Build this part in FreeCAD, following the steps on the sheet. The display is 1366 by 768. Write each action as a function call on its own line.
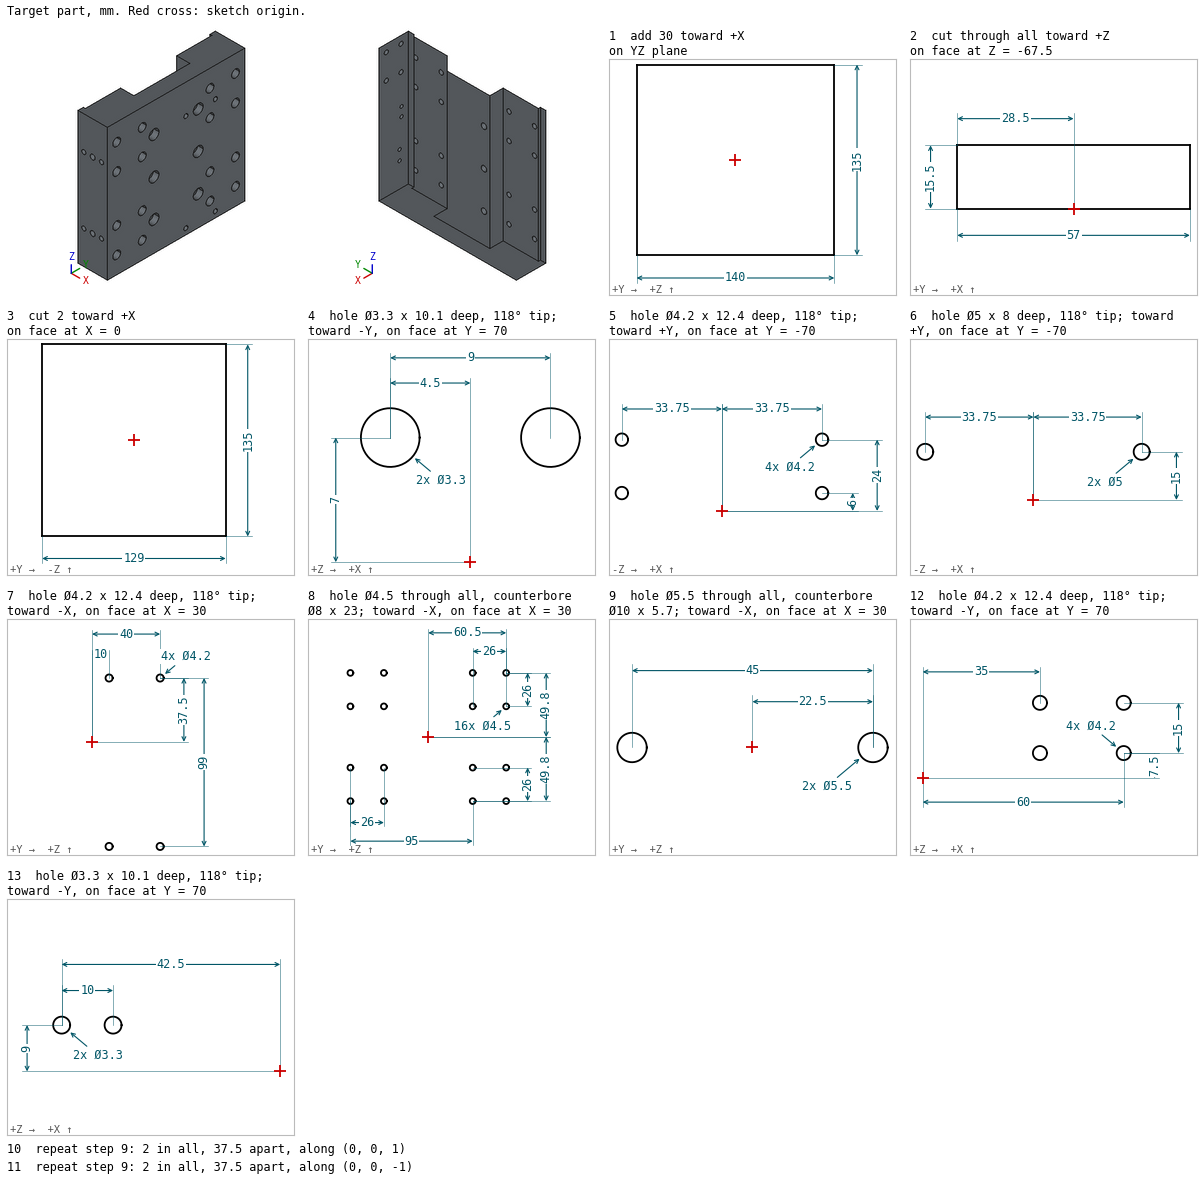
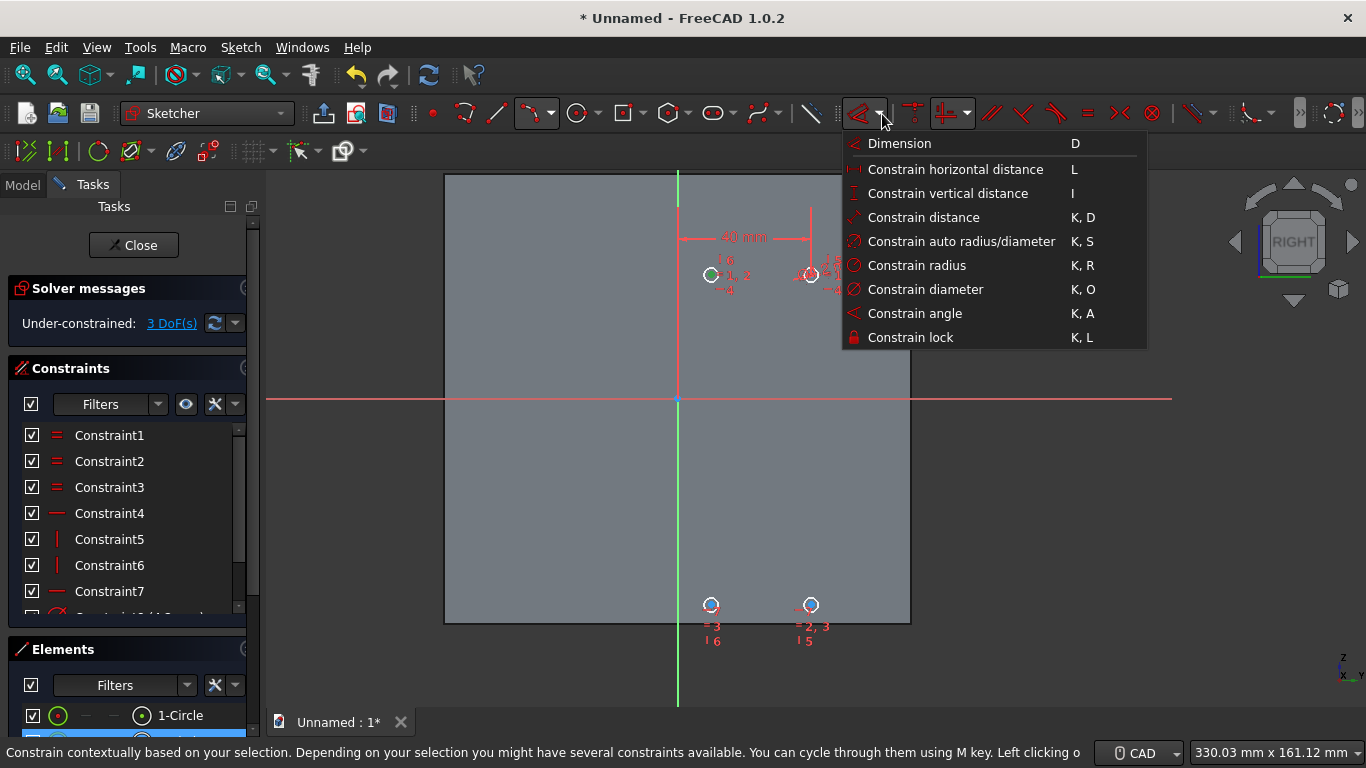
click(995, 169)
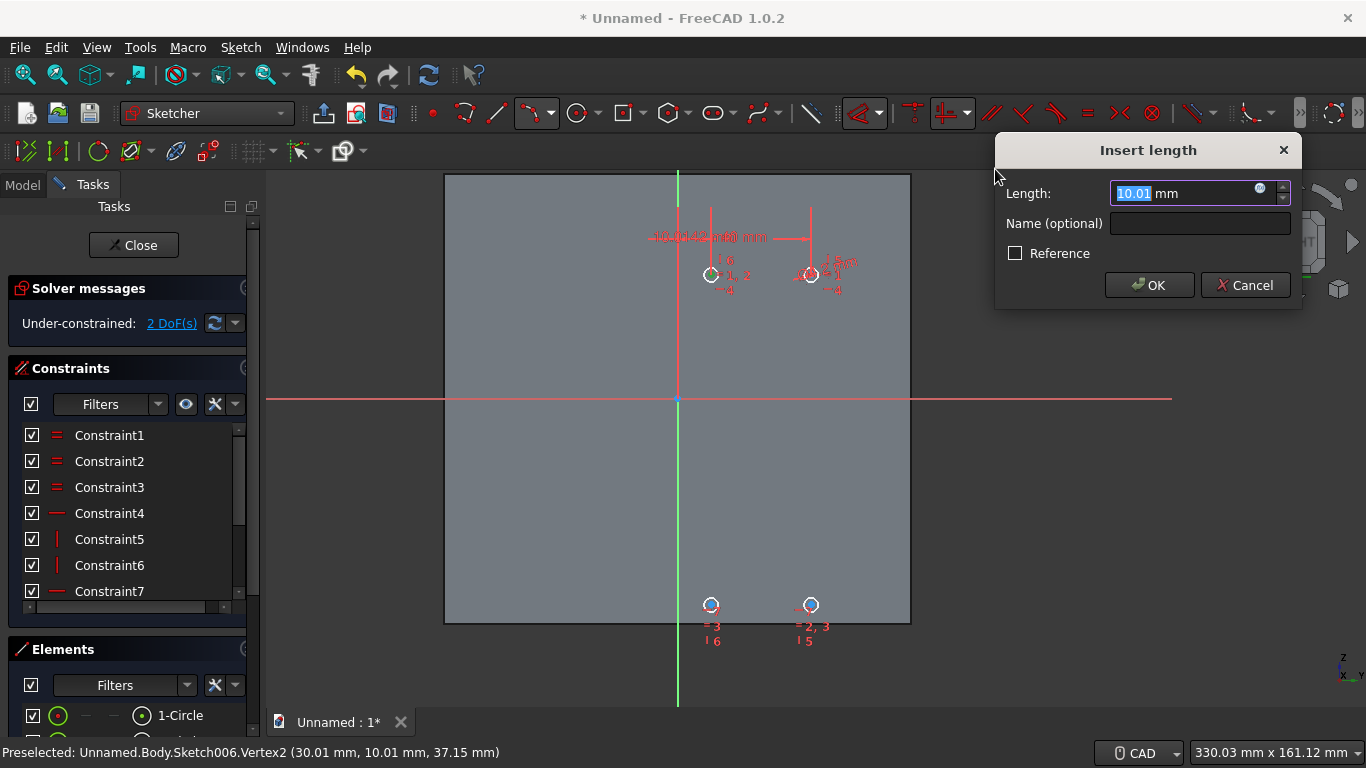
text(10)
key(Return)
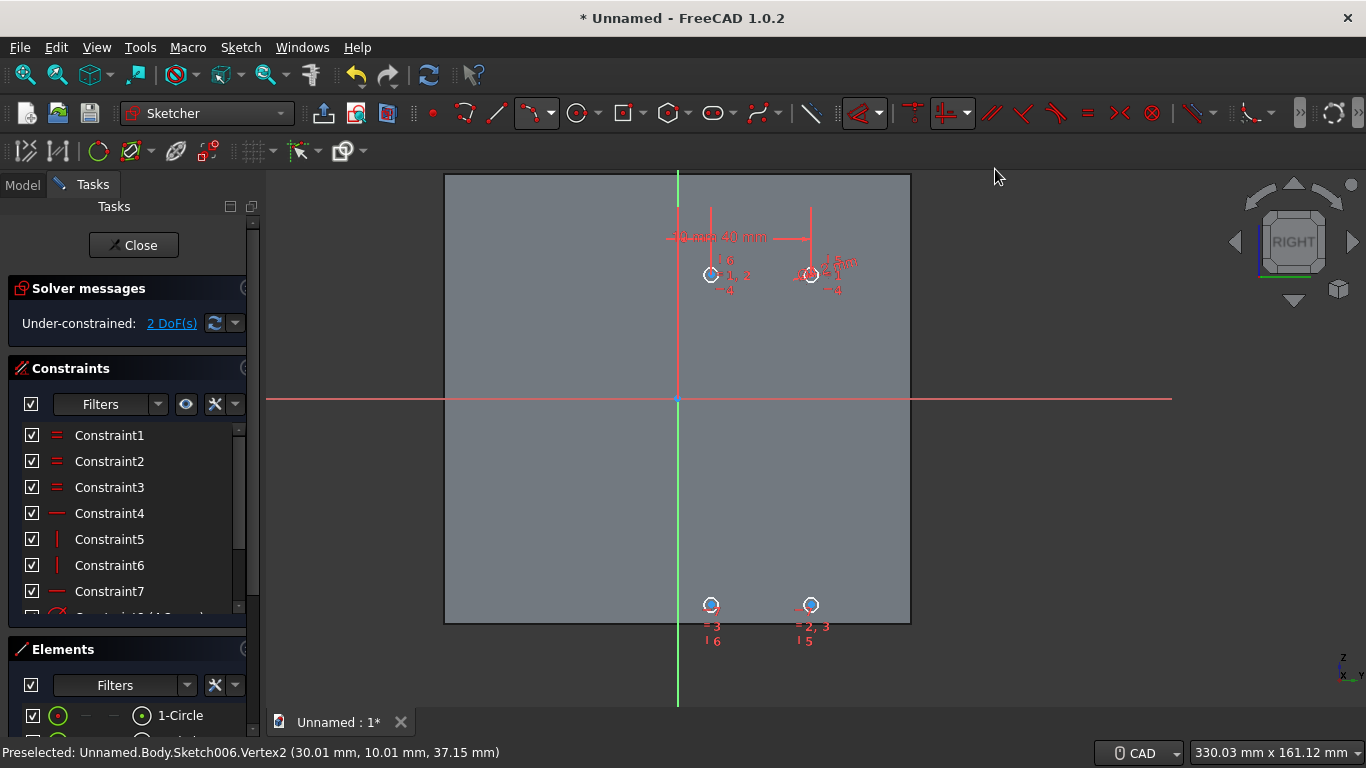
click(811, 275)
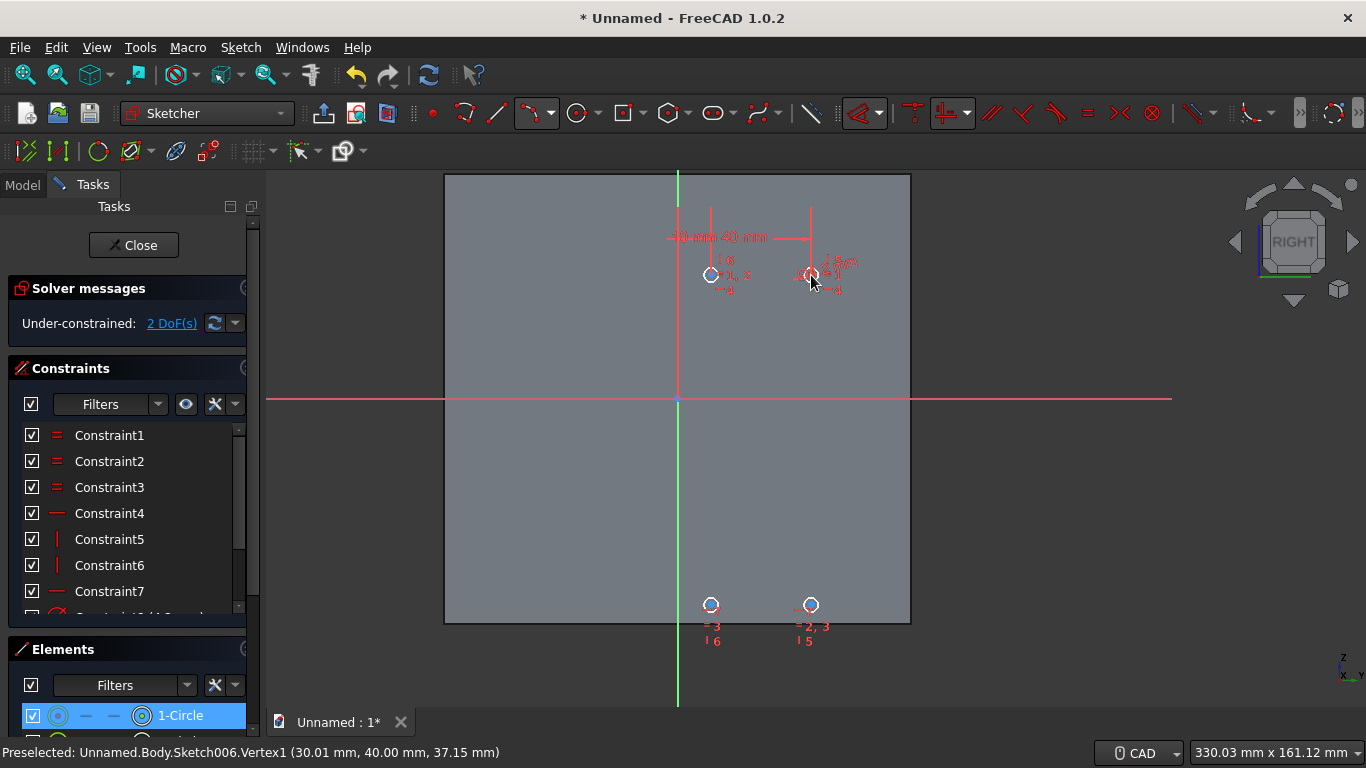
click(811, 605)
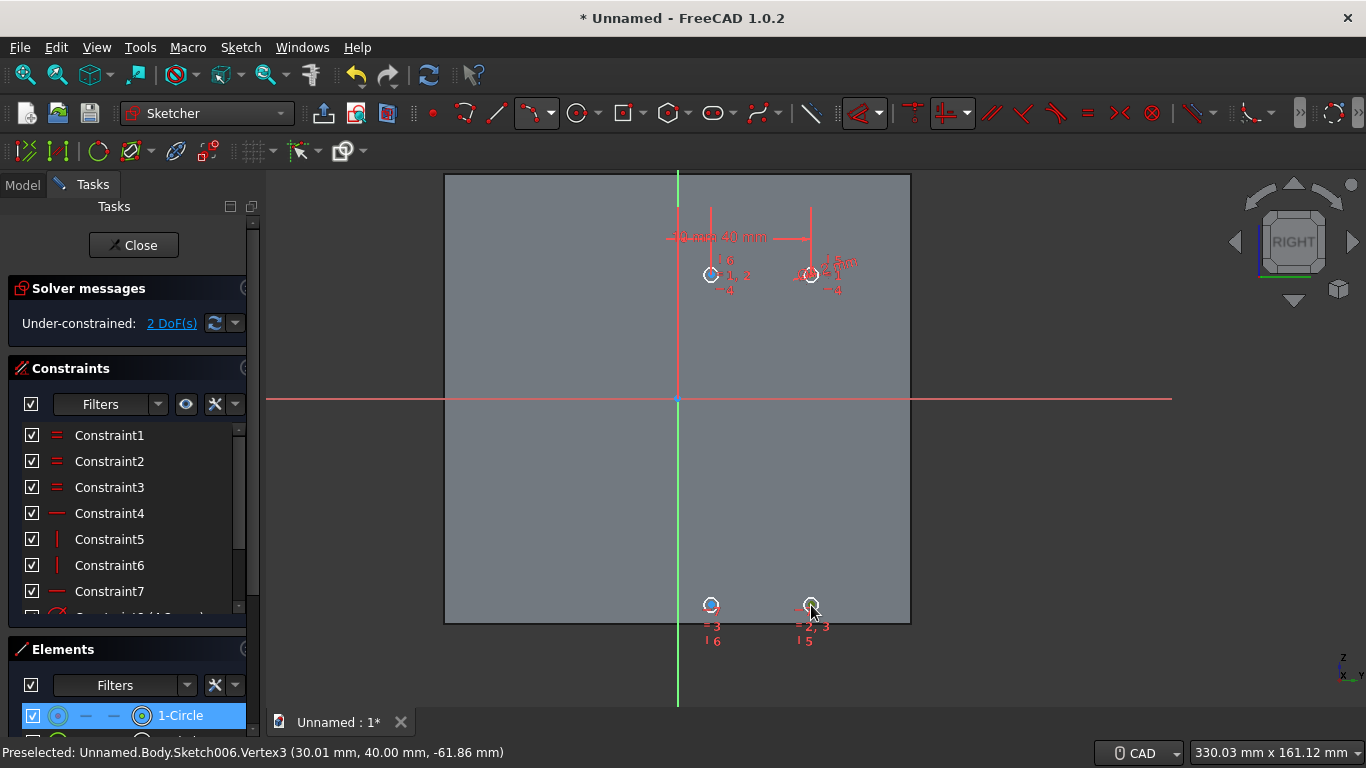
key(i)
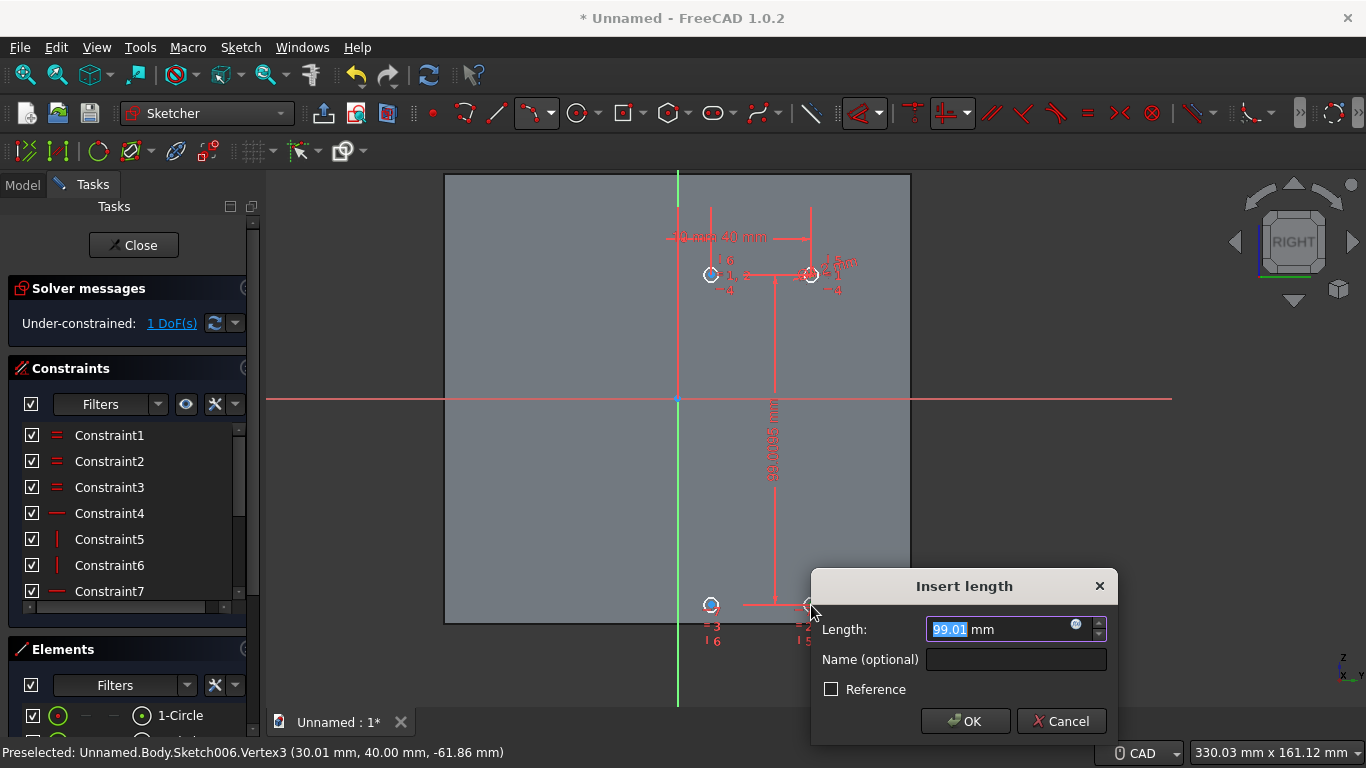
text(99)
key(Return)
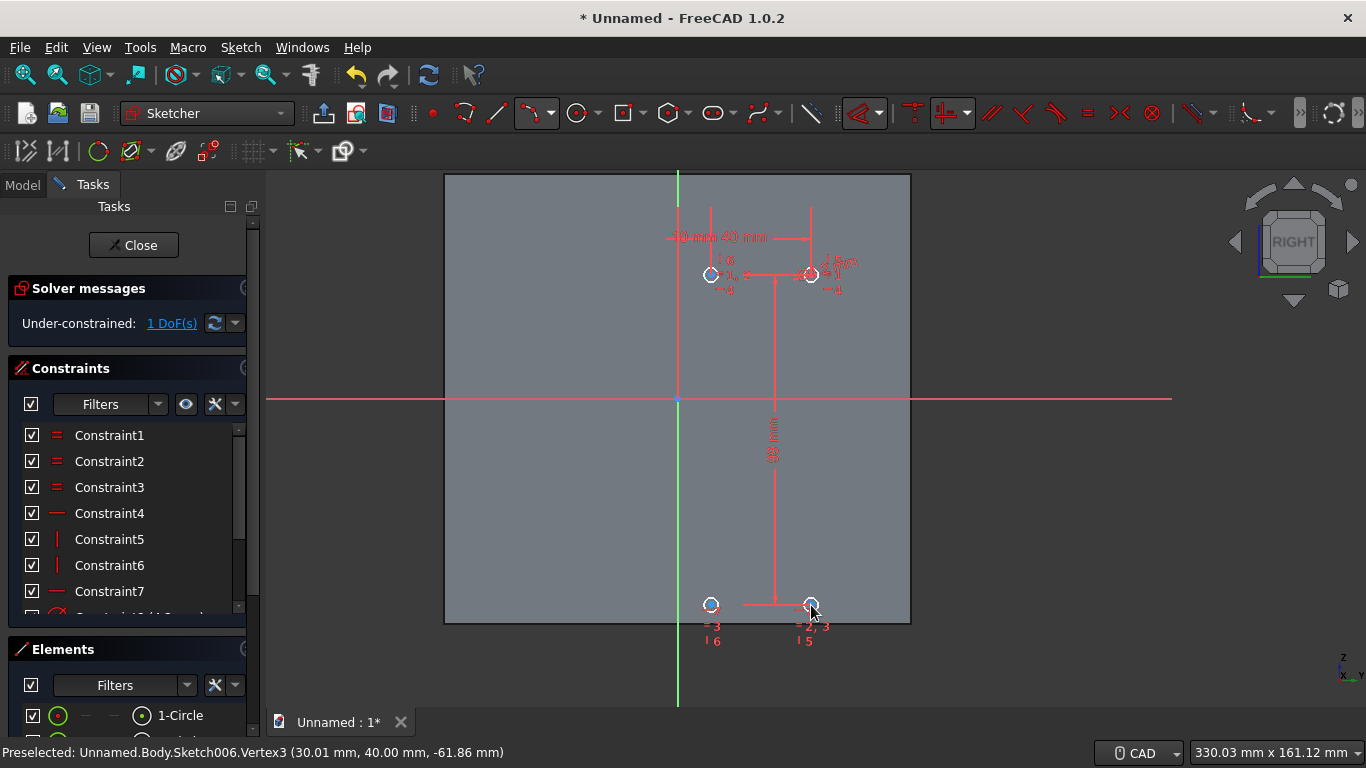
click(811, 275)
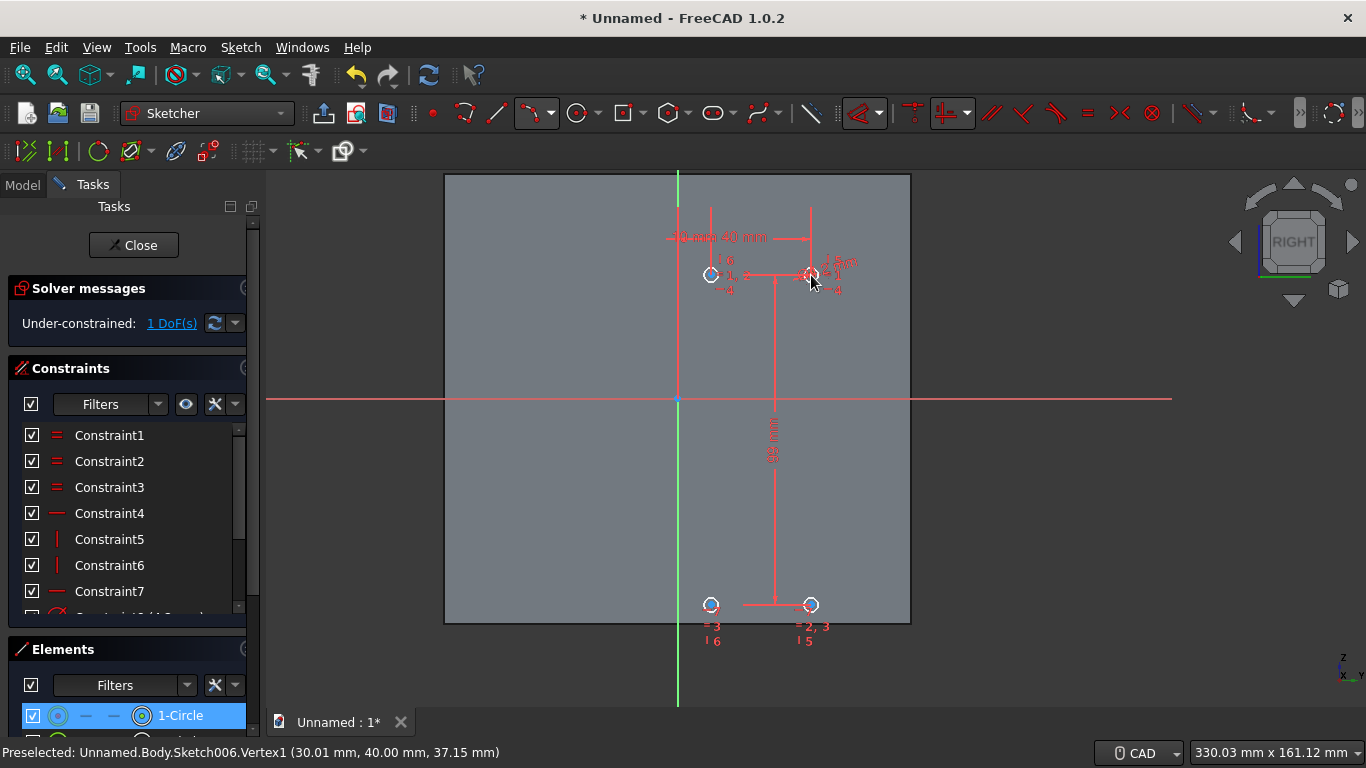
click(882, 114)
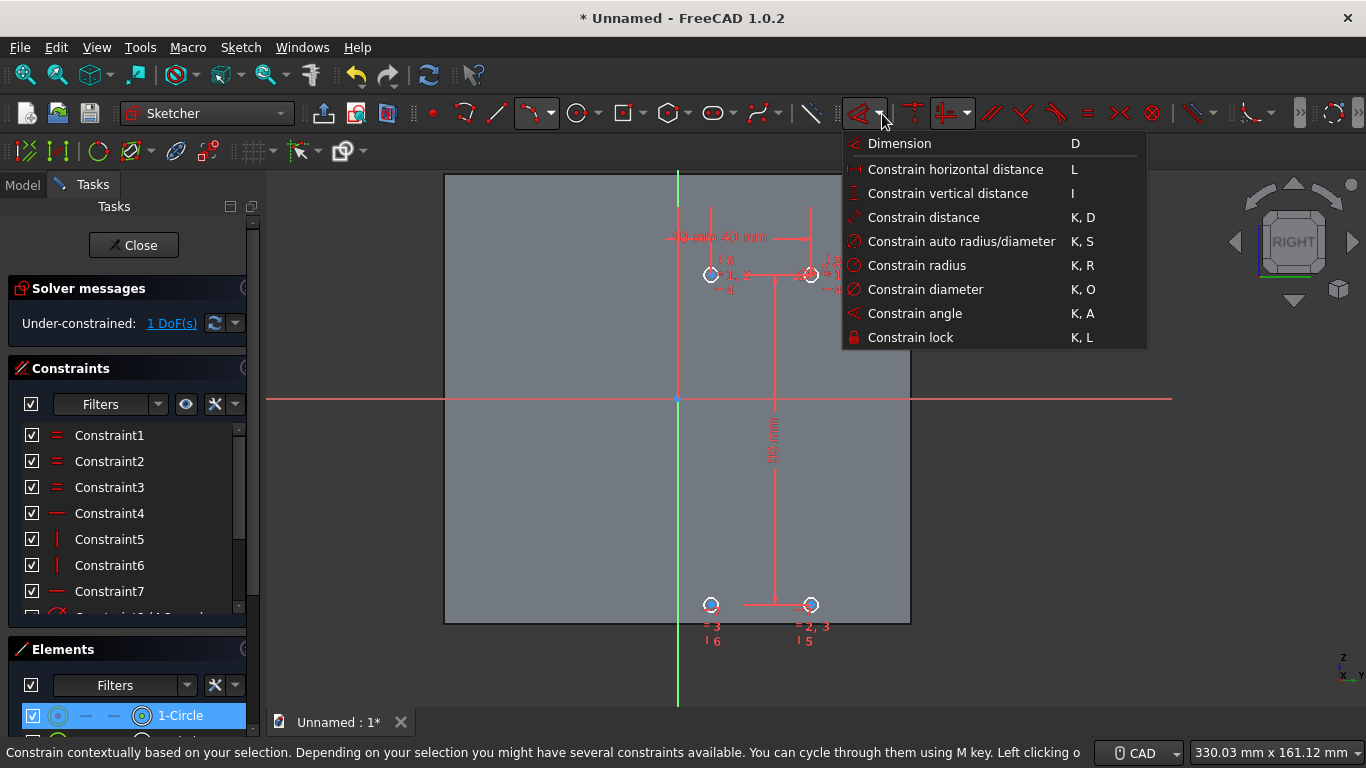
click(995, 193)